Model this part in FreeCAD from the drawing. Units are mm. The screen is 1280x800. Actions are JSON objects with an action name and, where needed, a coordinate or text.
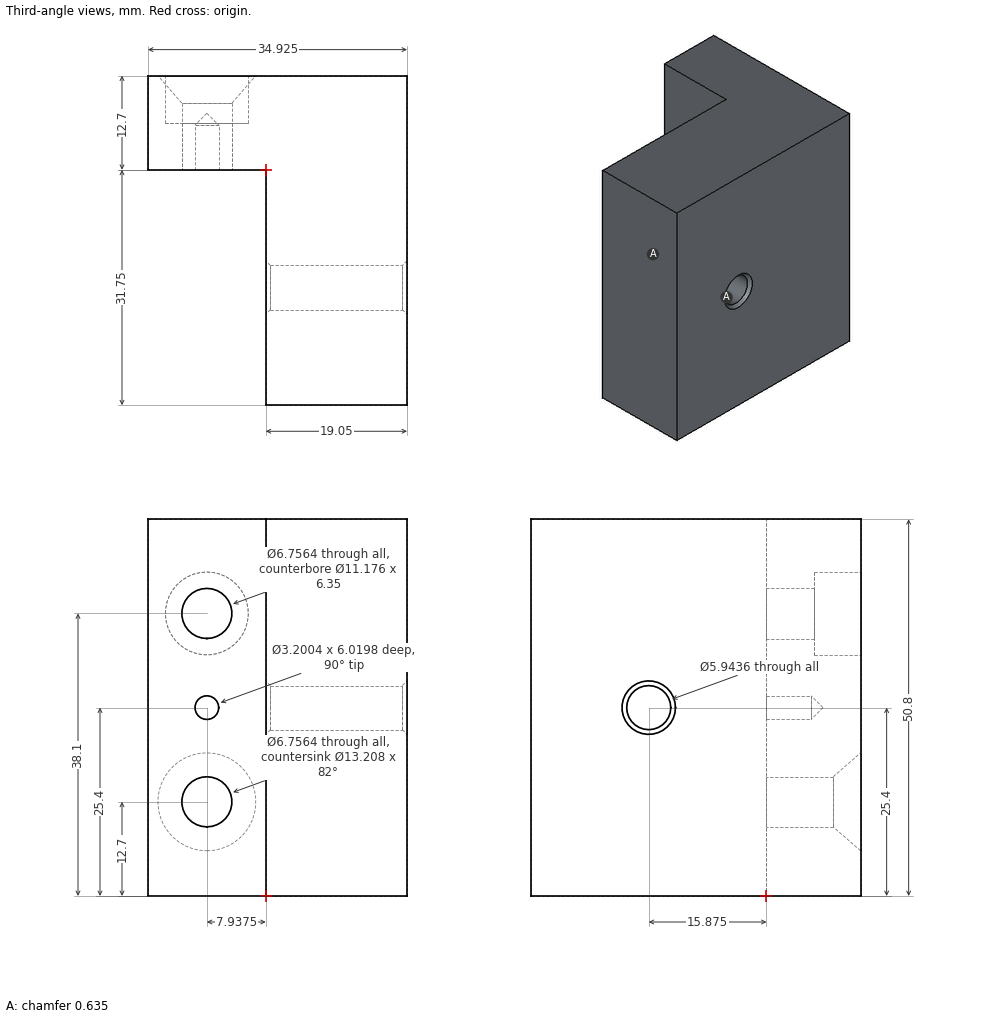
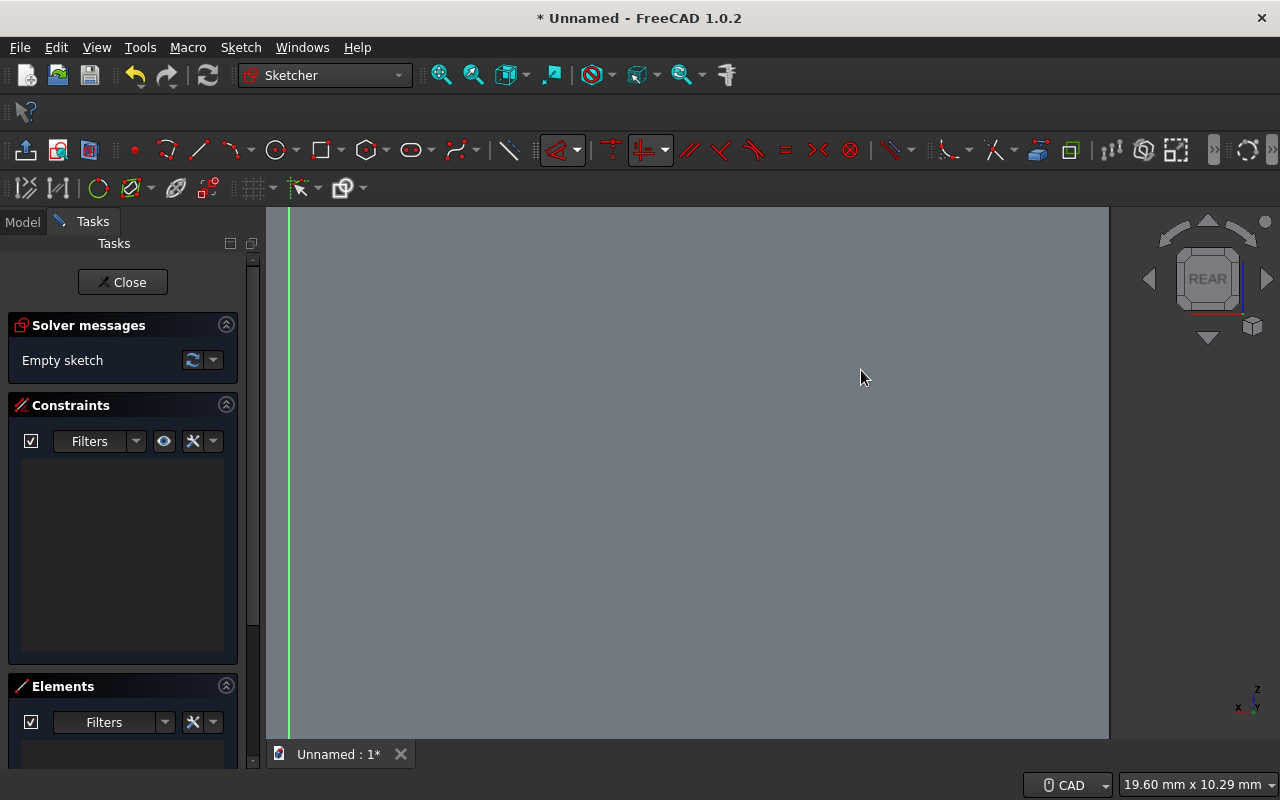
{"action": "left_click", "coordinate": [276, 150]}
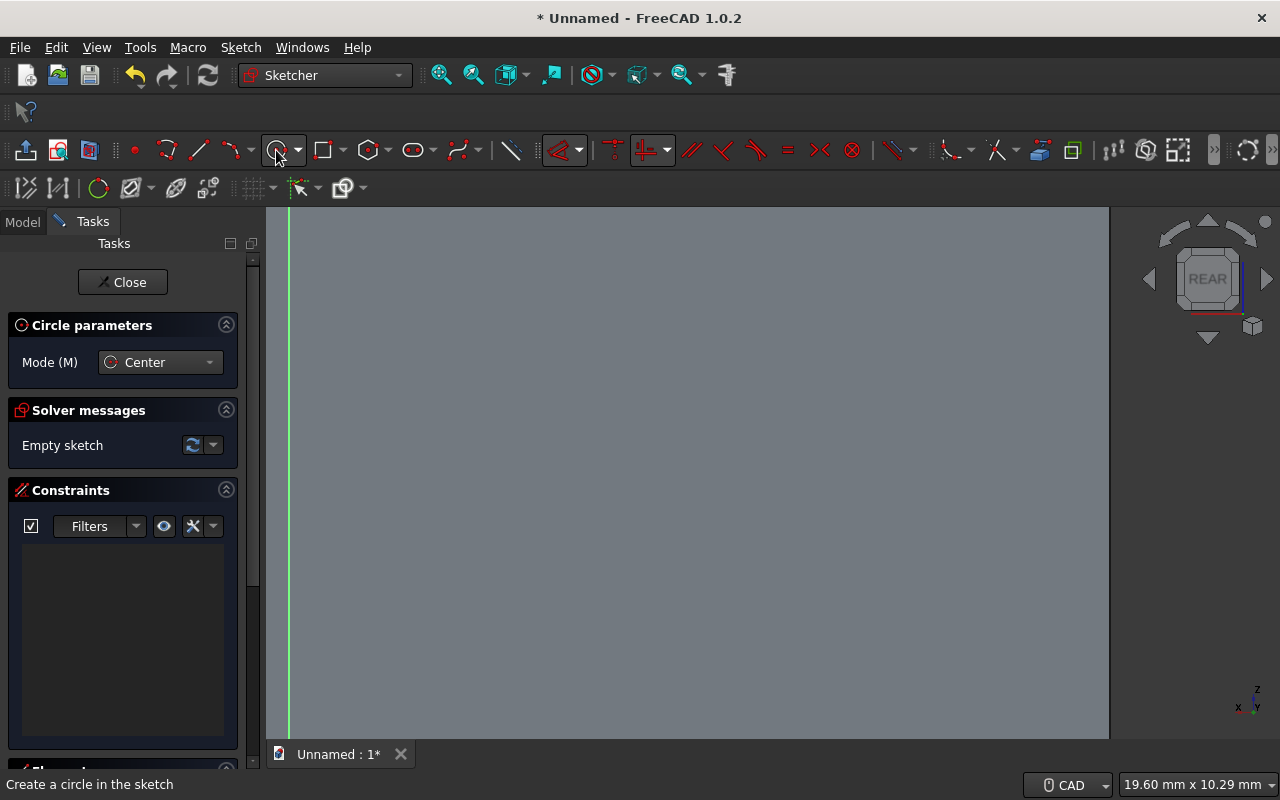
{"action": "left_click", "coordinate": [700, 472]}
{"action": "mouse_move", "coordinate": [823, 349]}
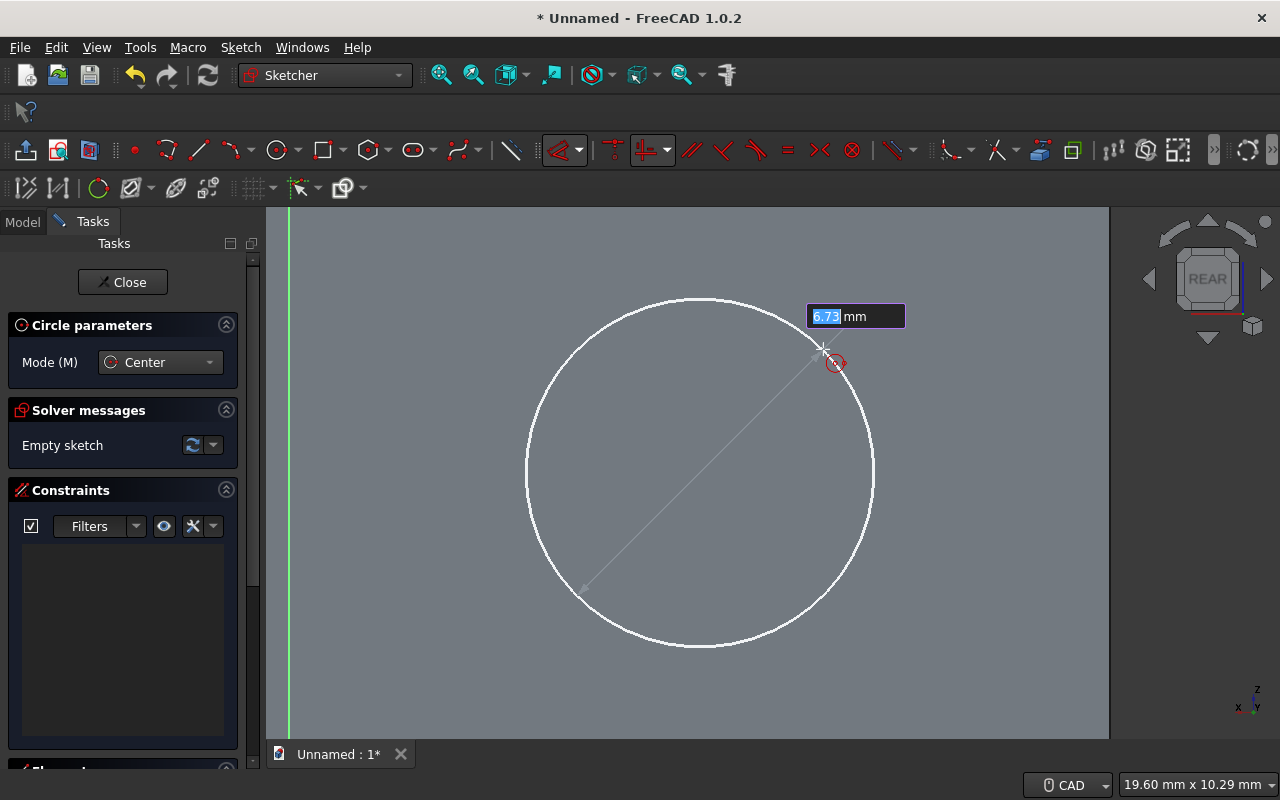
{"action": "type", "text": "6.7564"}
{"action": "key", "text": "Return"}
{"action": "key", "text": "Escape"}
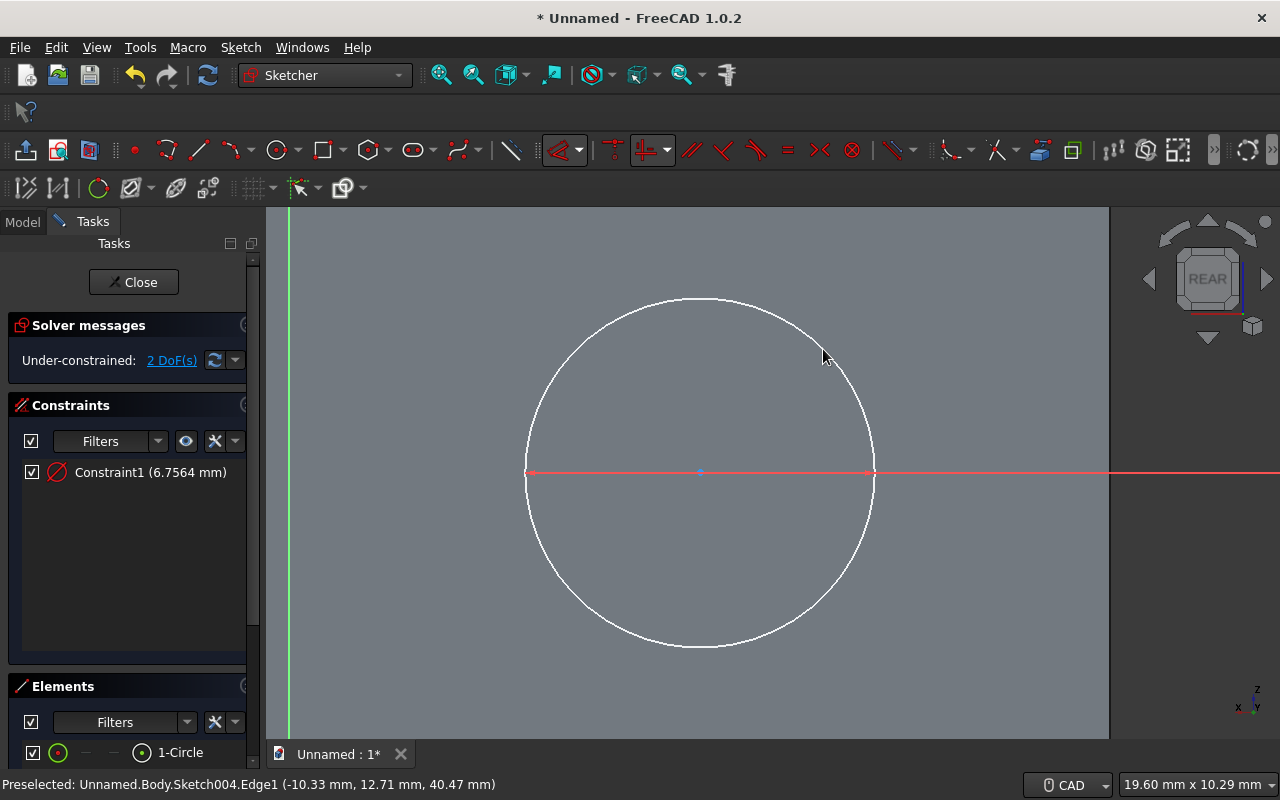
{"action": "left_click", "coordinate": [700, 473]}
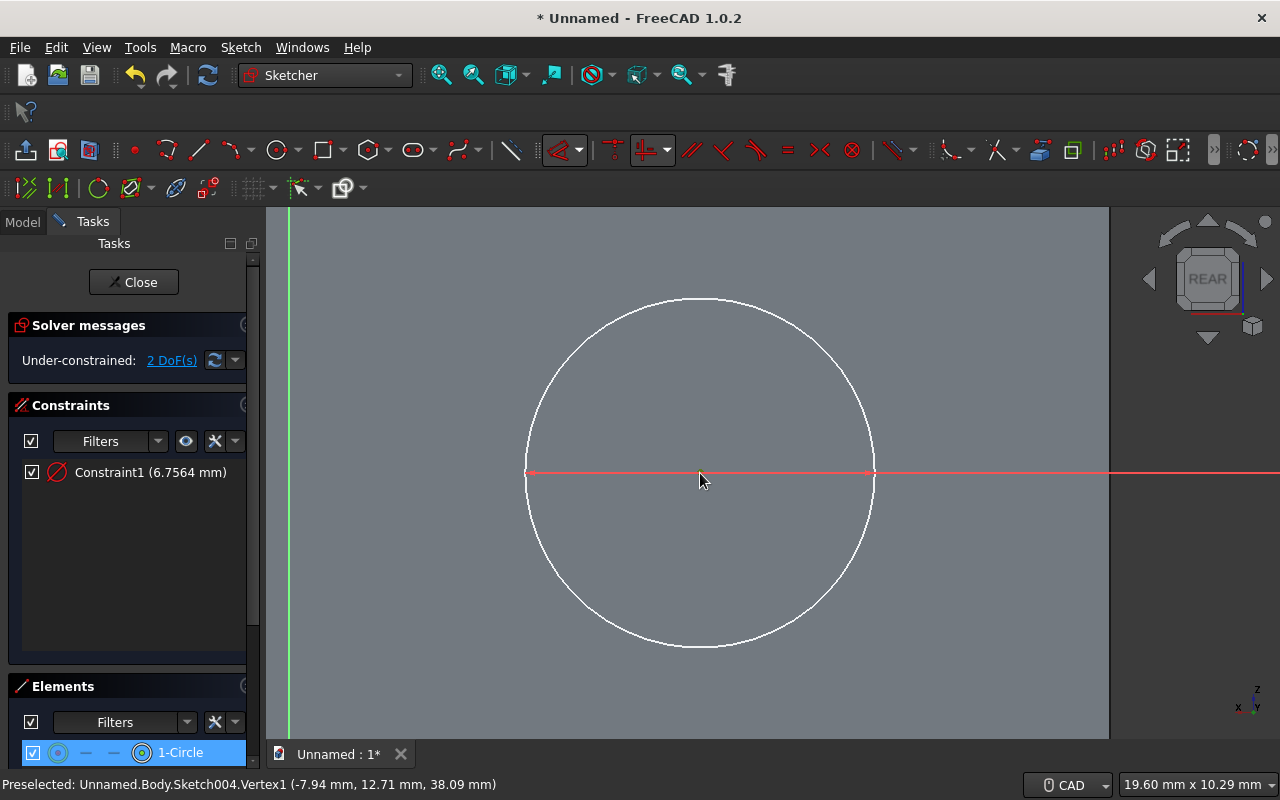
{"action": "left_click", "coordinate": [582, 150]}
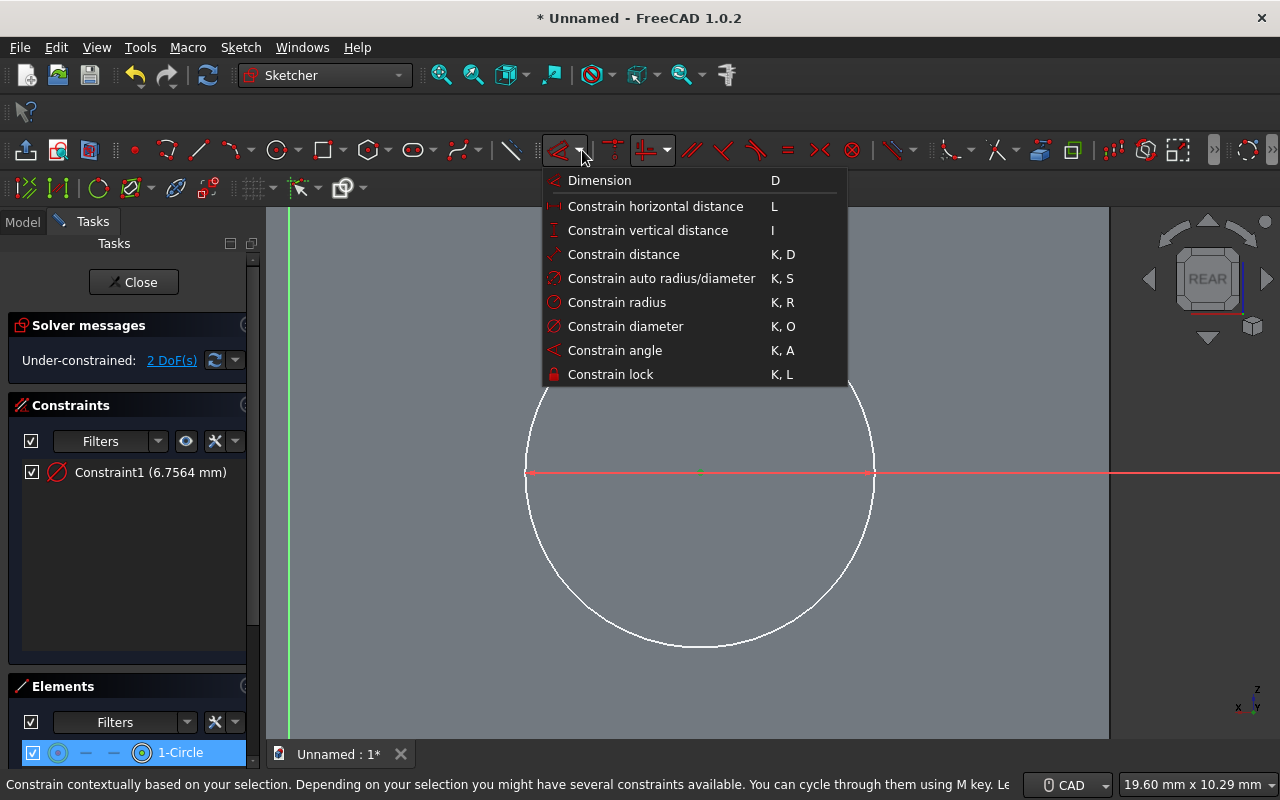
{"action": "left_click", "coordinate": [695, 230]}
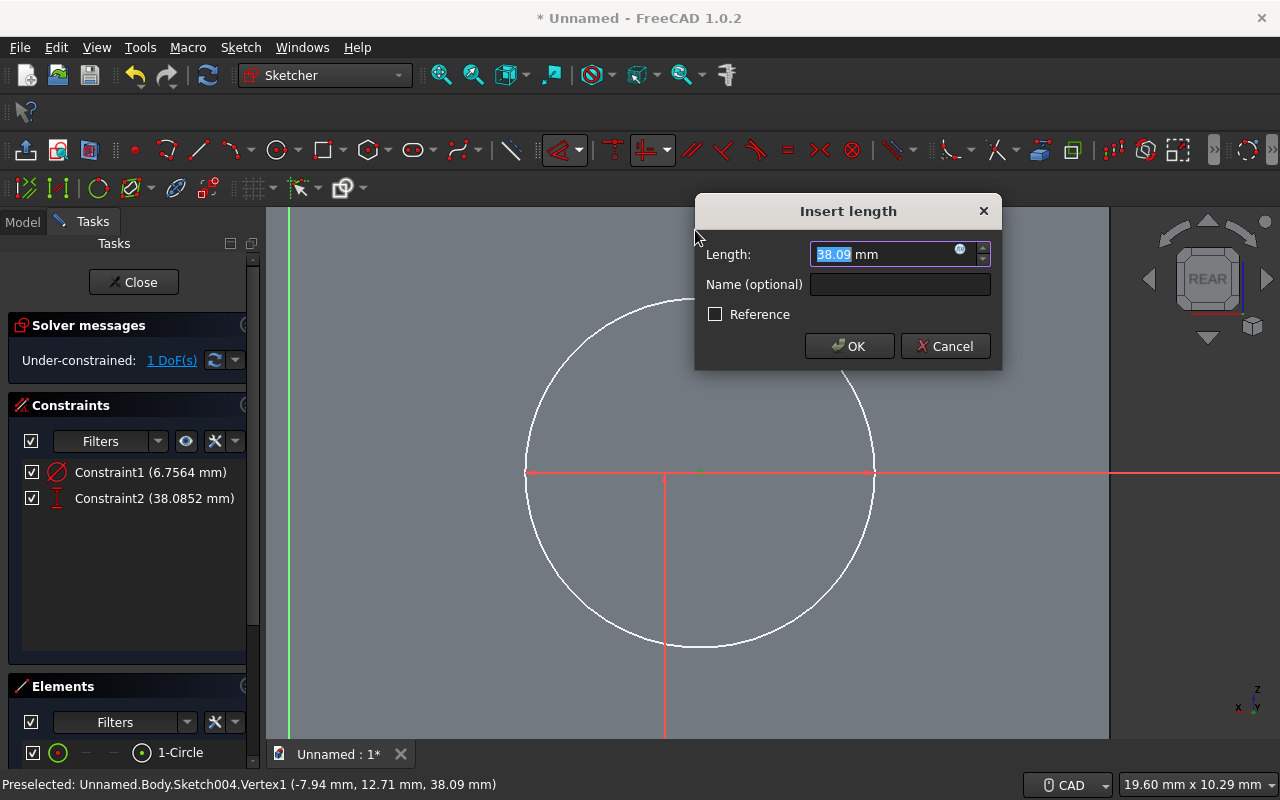
{"action": "type", "text": "38.1"}
{"action": "key", "text": "Return"}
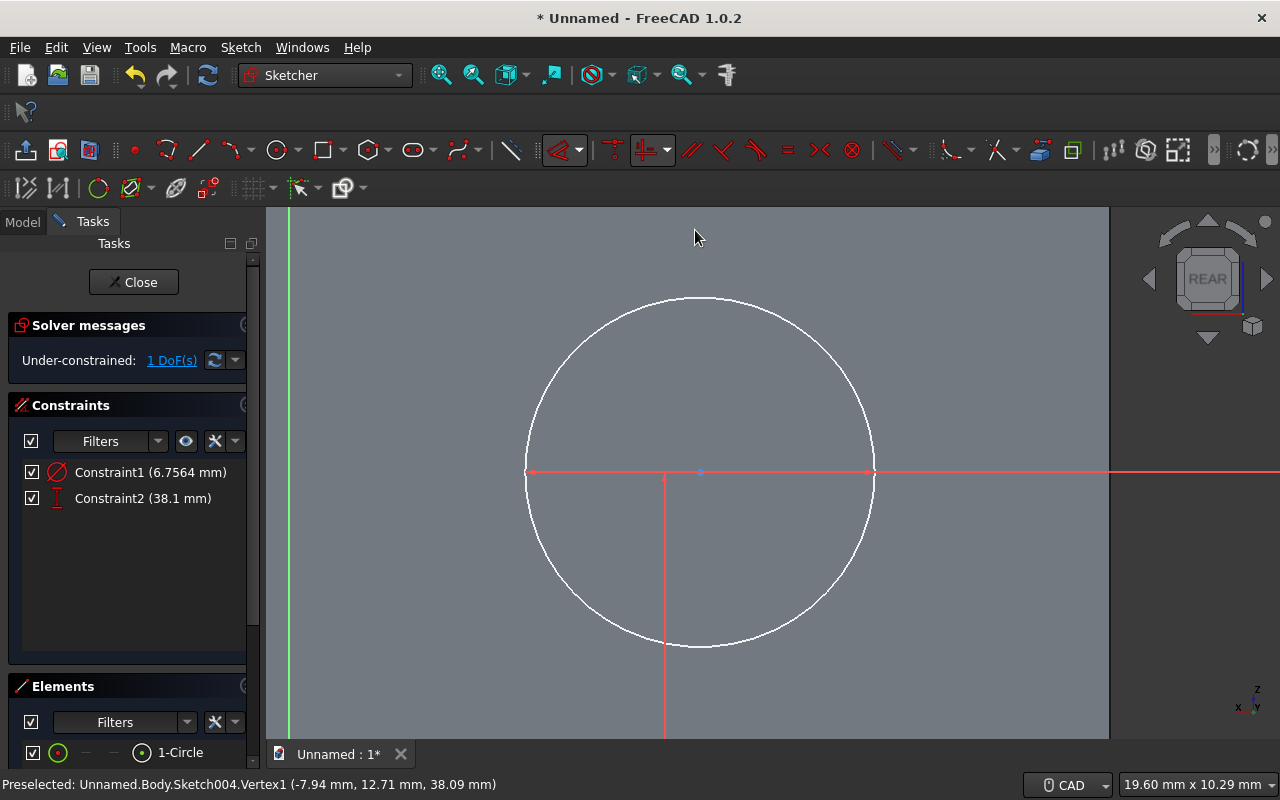
{"action": "left_click", "coordinate": [700, 472]}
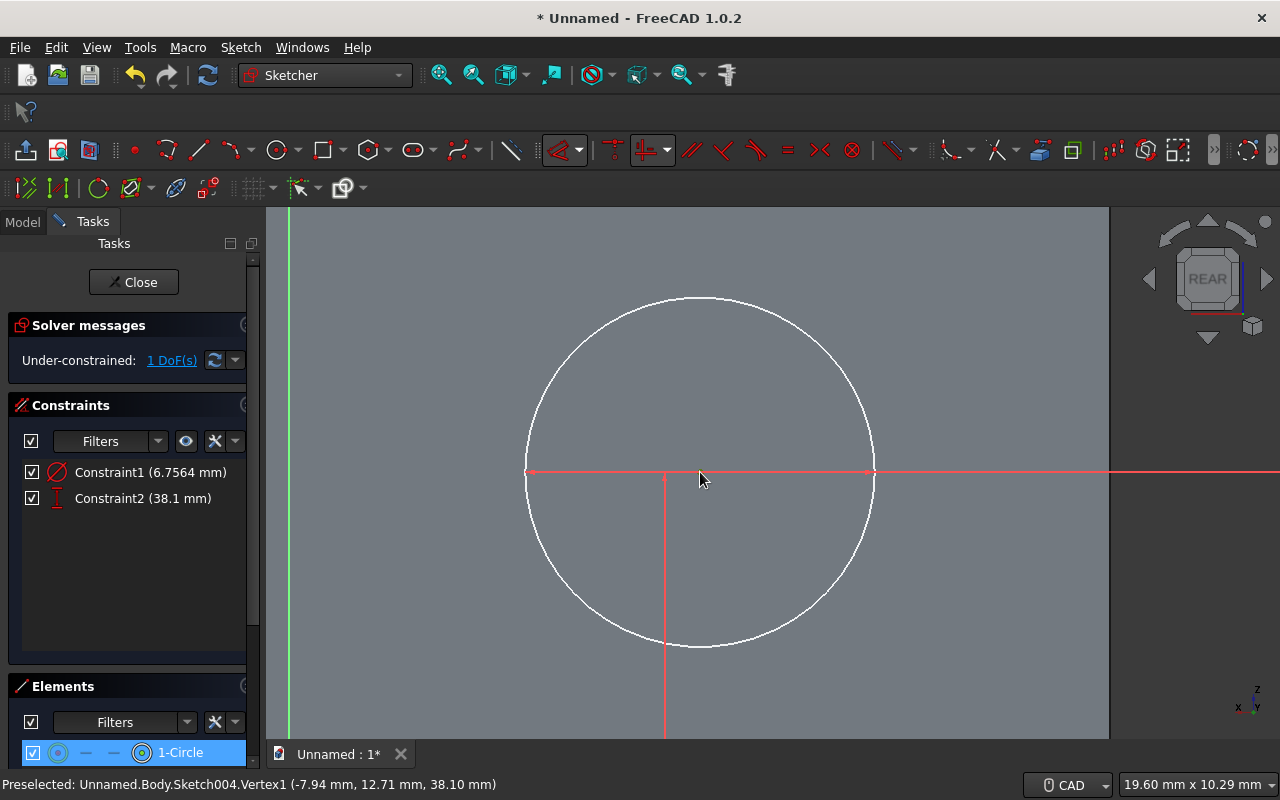
{"action": "key", "text": "l"}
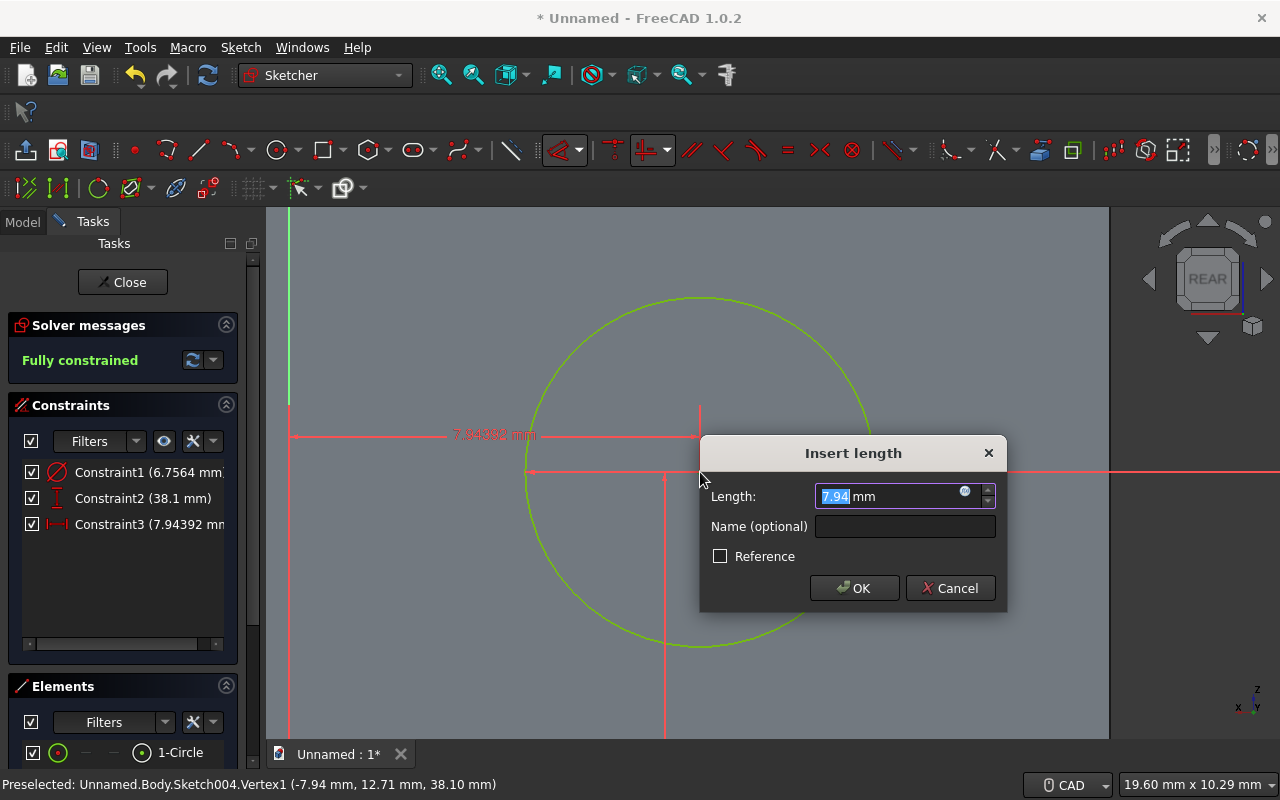
{"action": "type", "text": "7.9375"}
{"action": "key", "text": "Return"}